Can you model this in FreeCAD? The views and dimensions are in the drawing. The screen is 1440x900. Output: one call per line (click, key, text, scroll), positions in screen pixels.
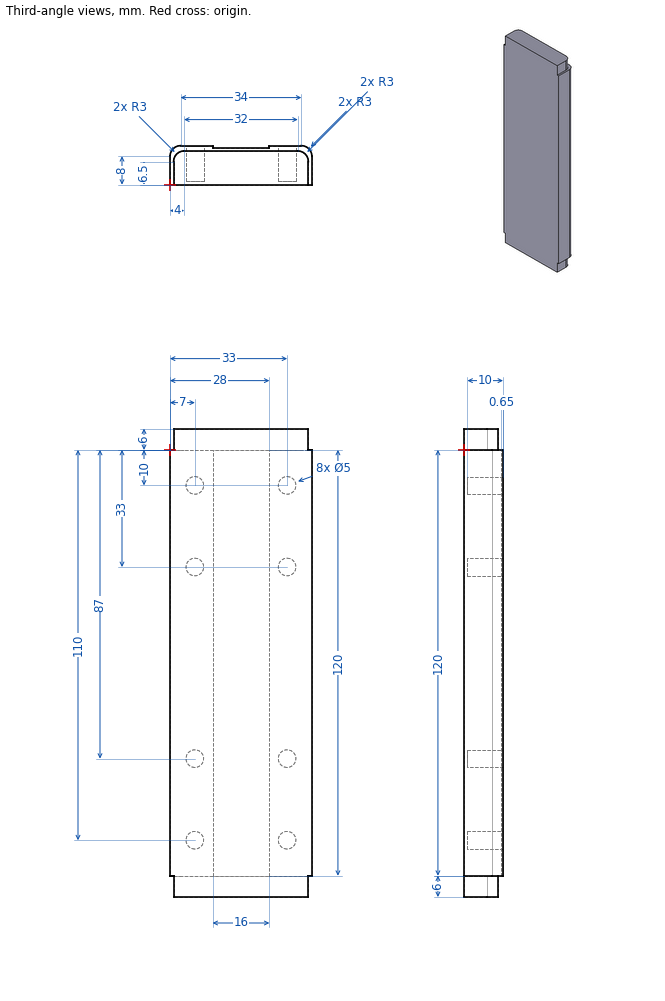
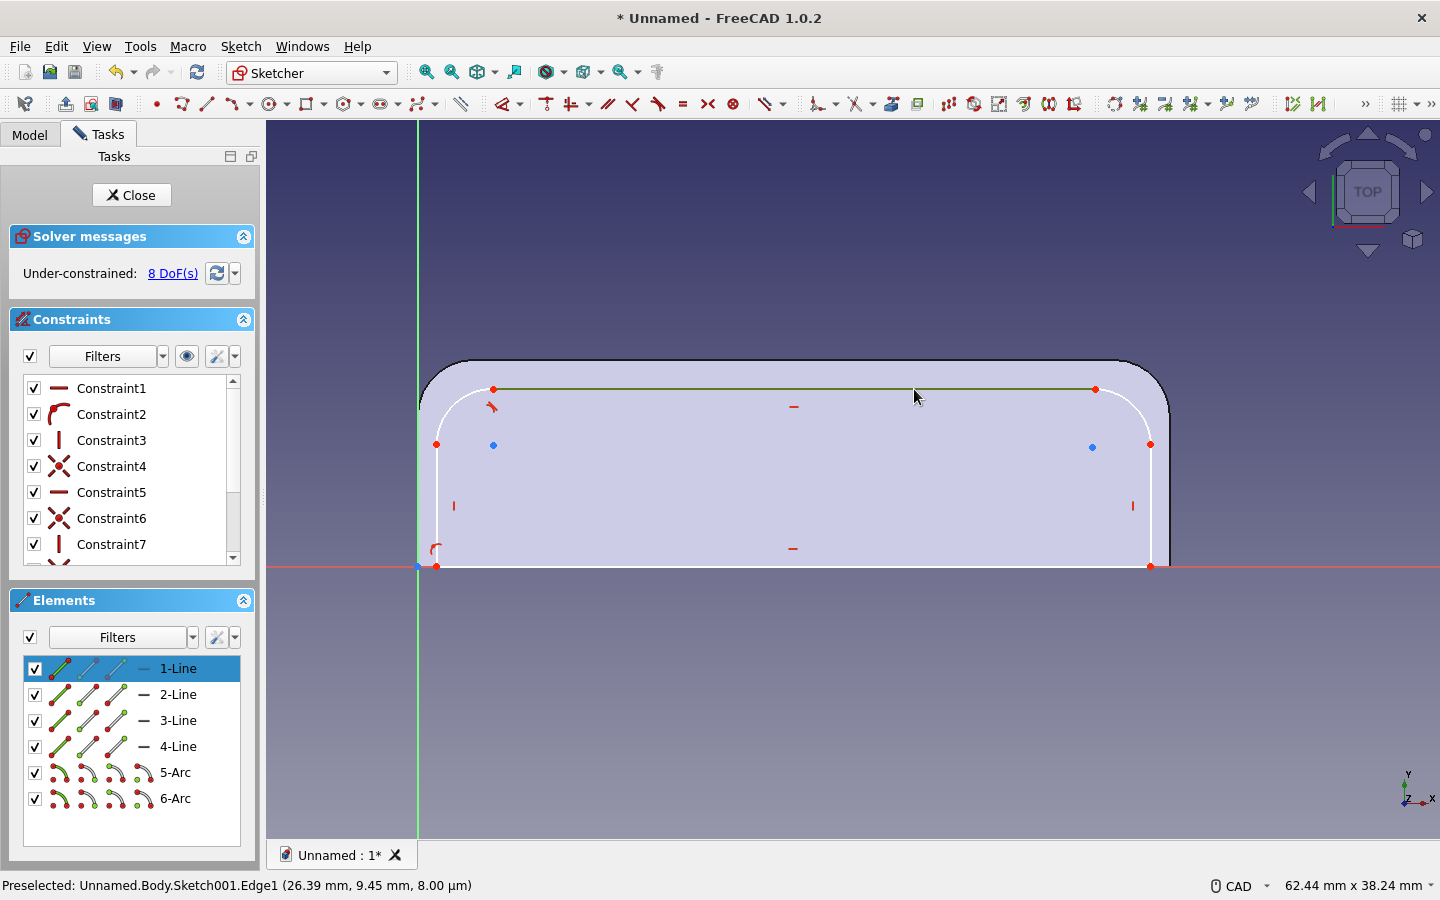
click(1144, 420)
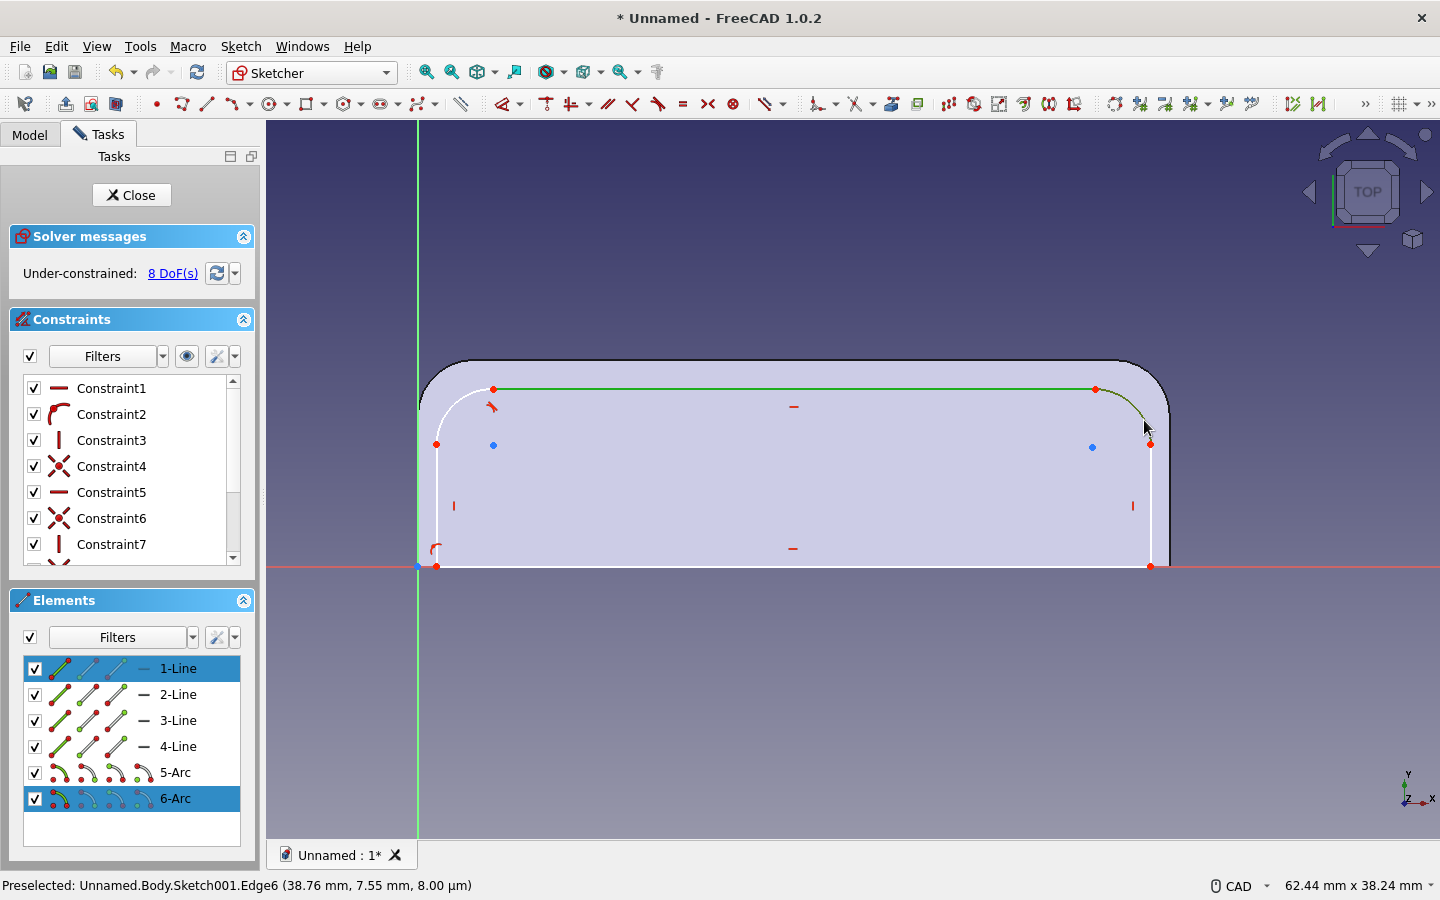
click(658, 104)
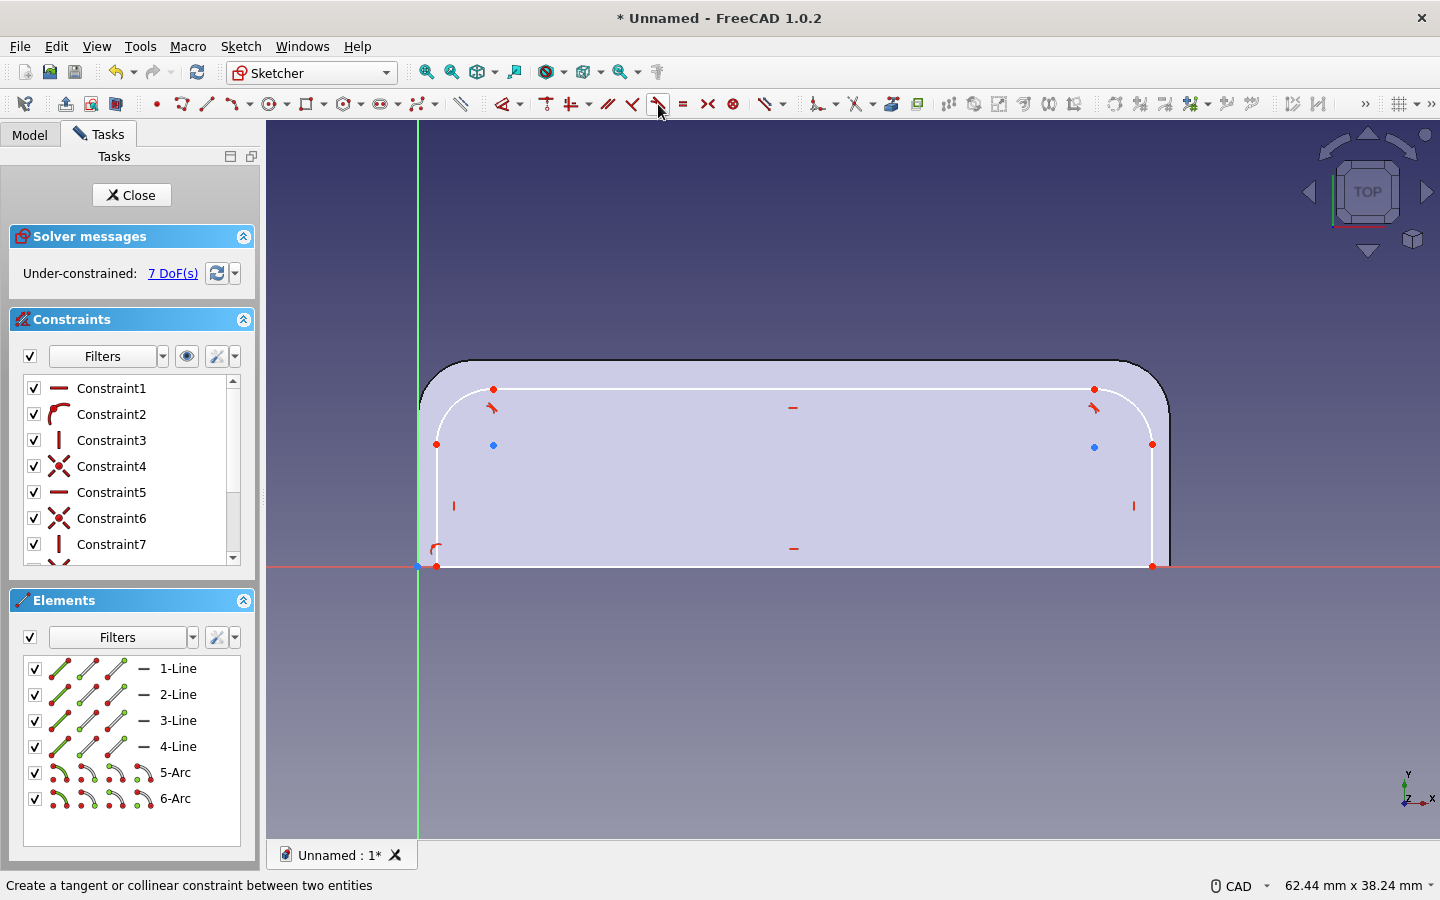
click(437, 481)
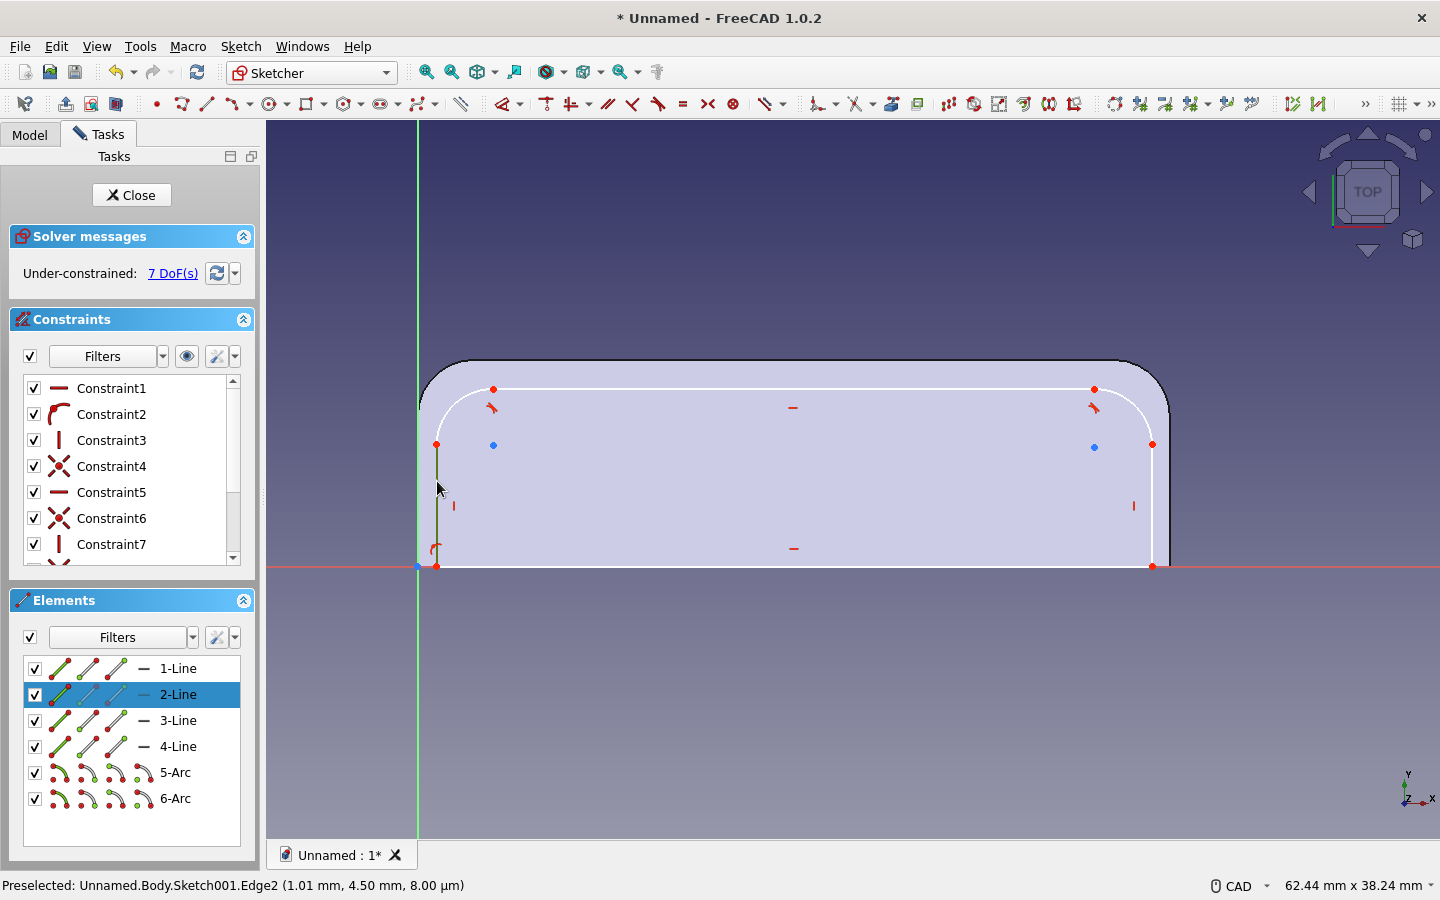
click(468, 395)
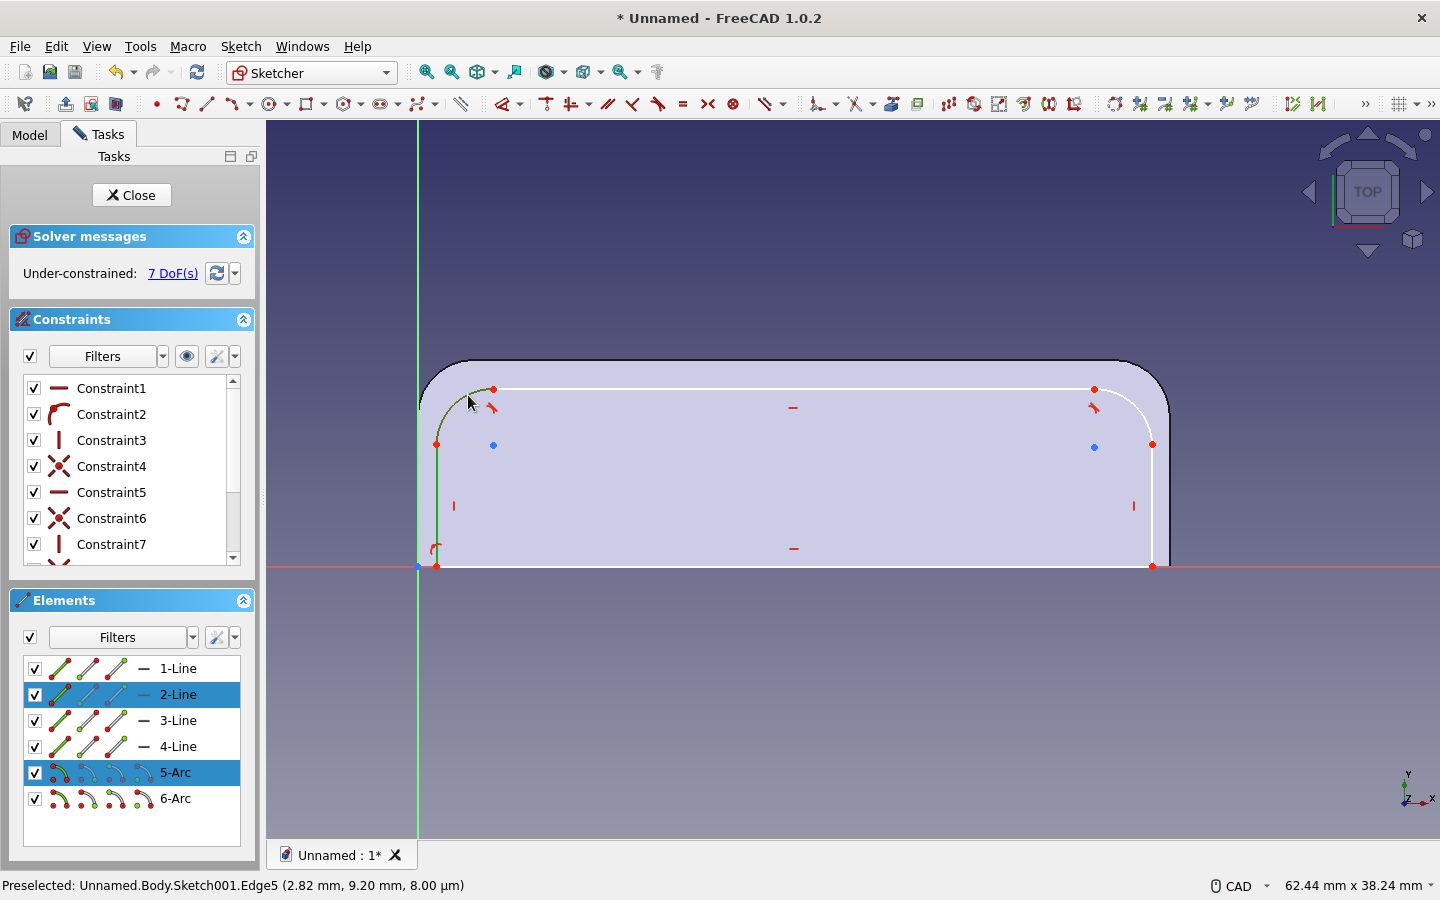
click(658, 104)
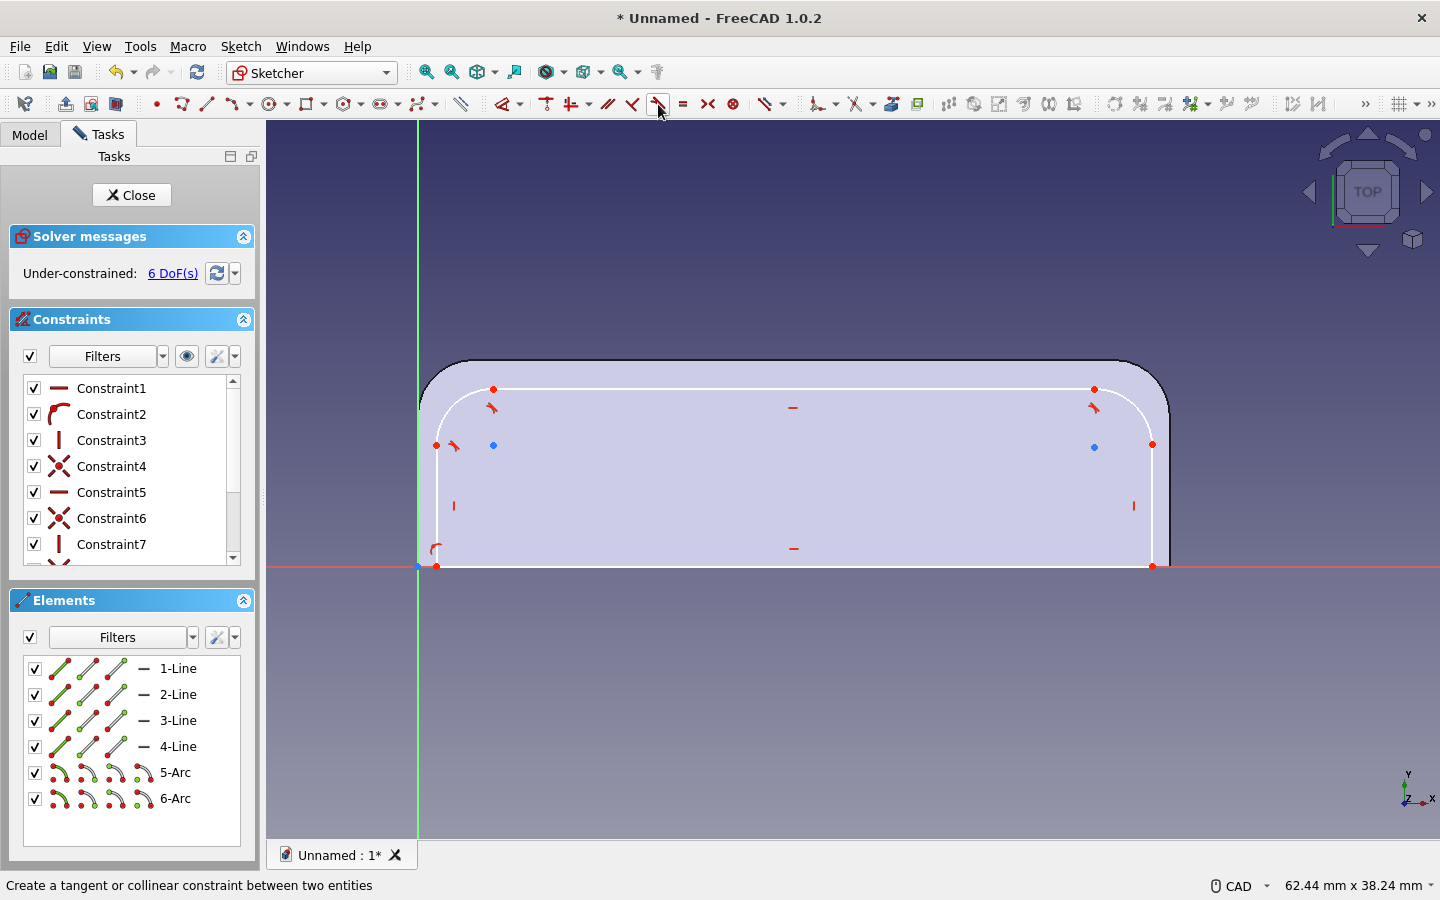
click(1152, 530)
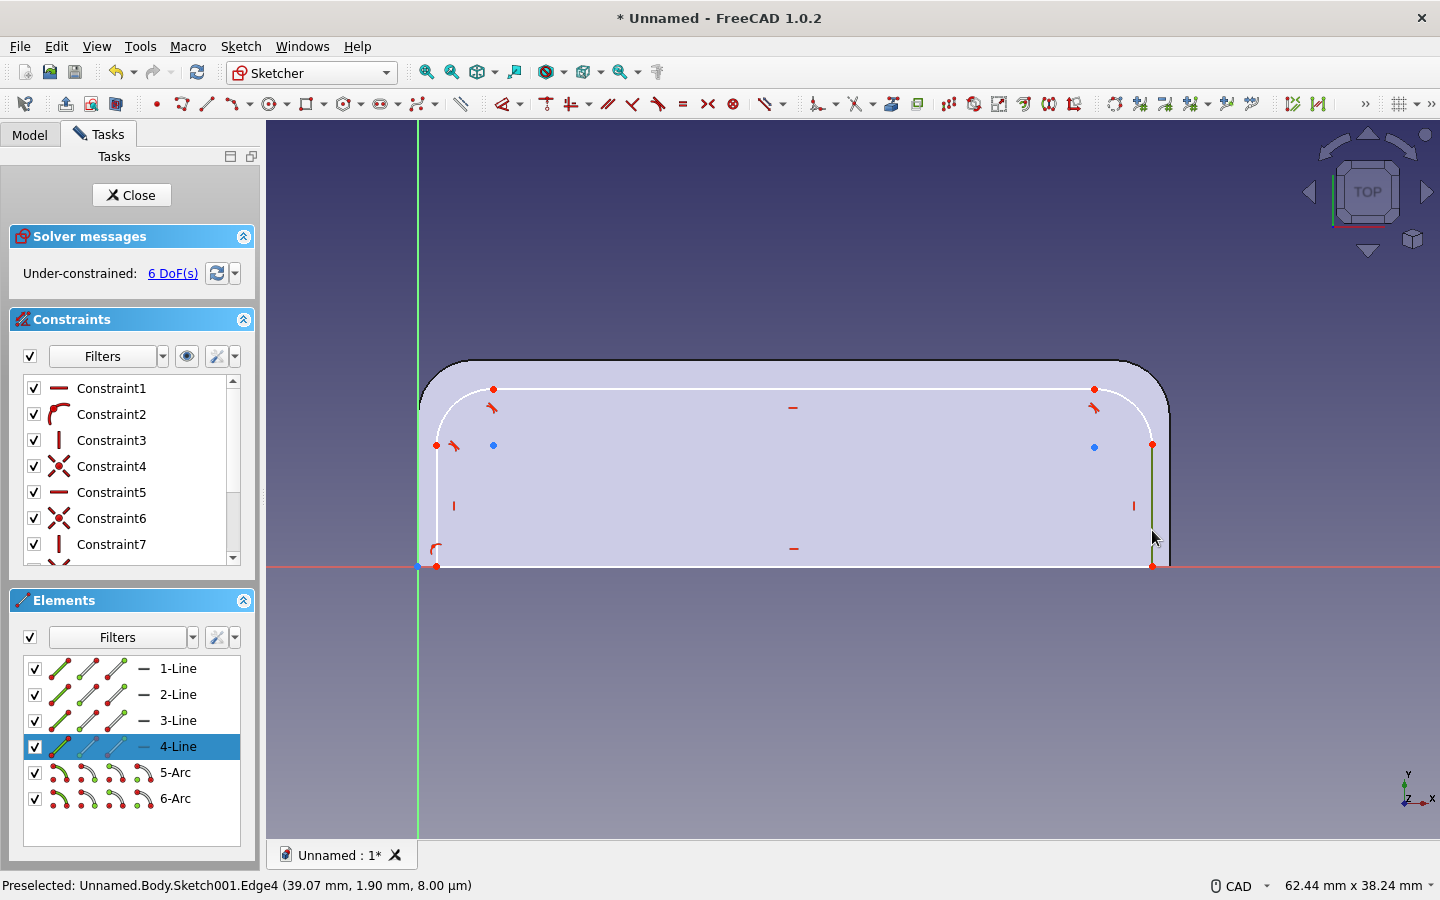
click(1145, 419)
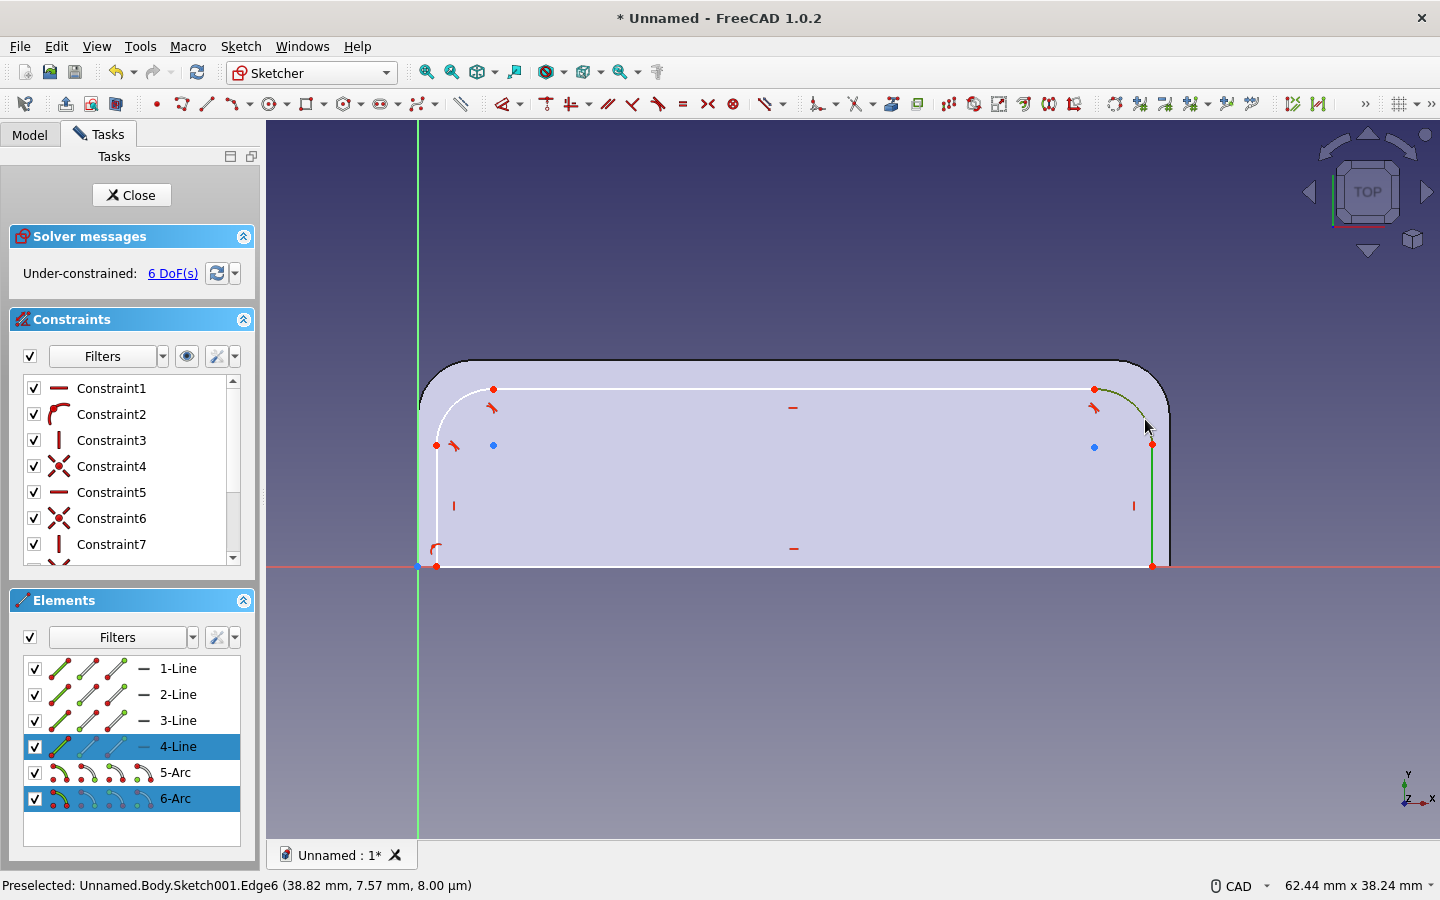
click(658, 104)